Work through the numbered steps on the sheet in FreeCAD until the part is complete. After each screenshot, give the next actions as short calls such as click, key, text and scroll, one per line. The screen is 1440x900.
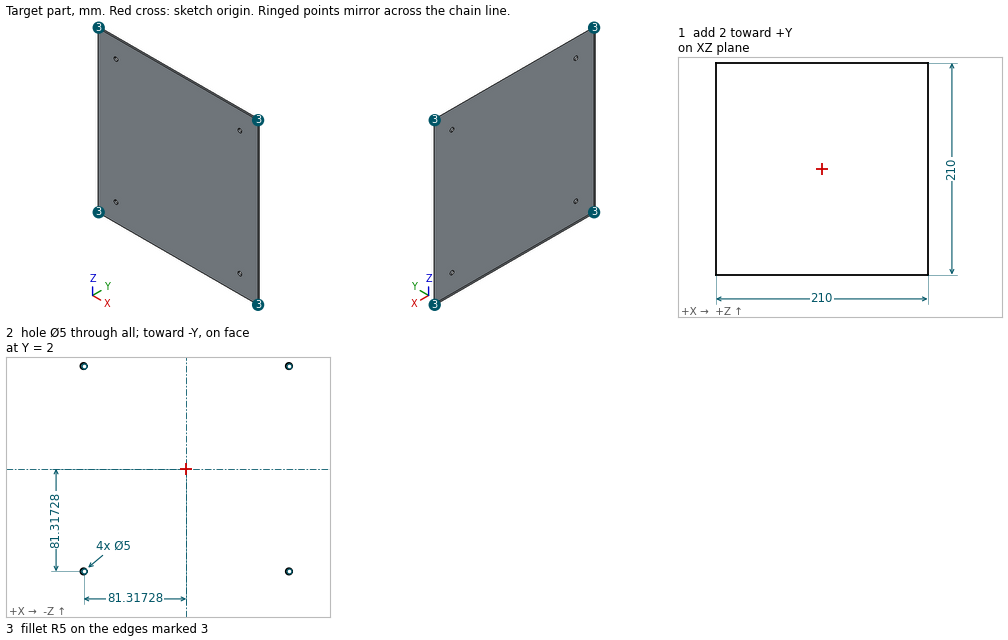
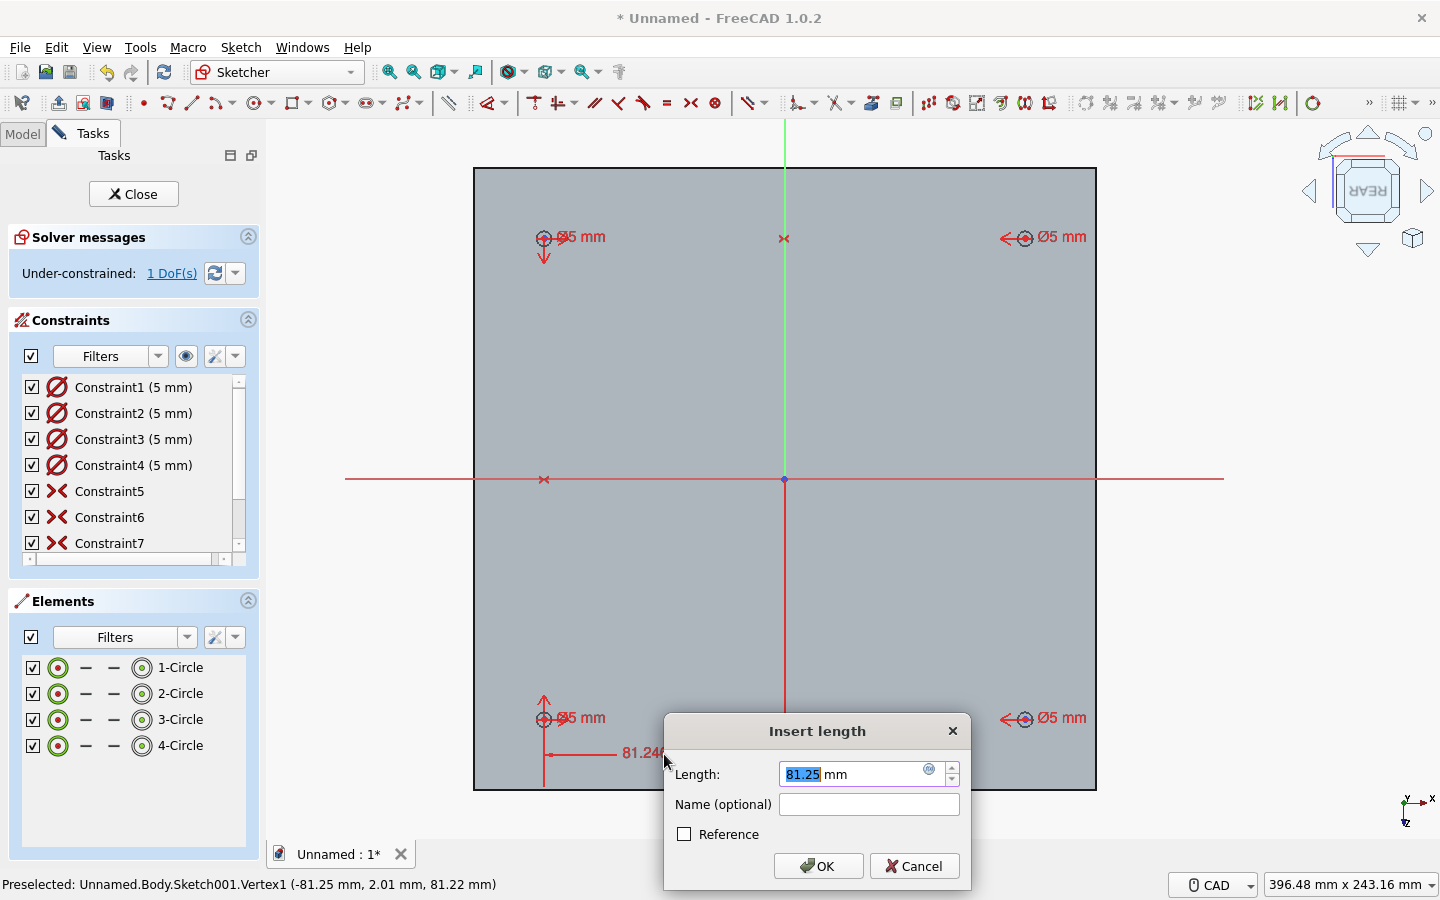
text(81.31728)
key(Return)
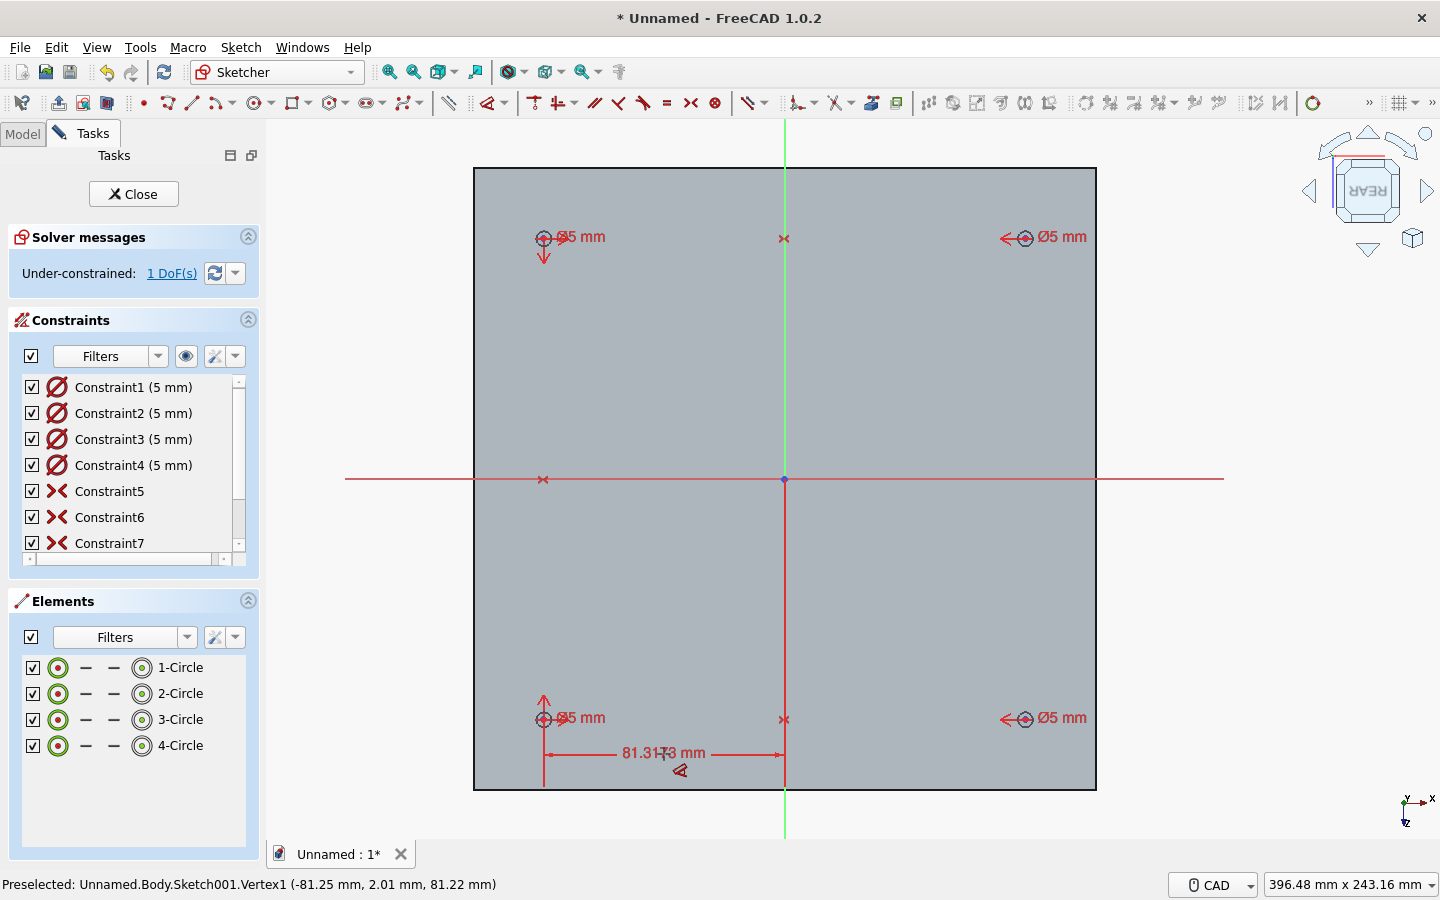
click(544, 720)
click(510, 600)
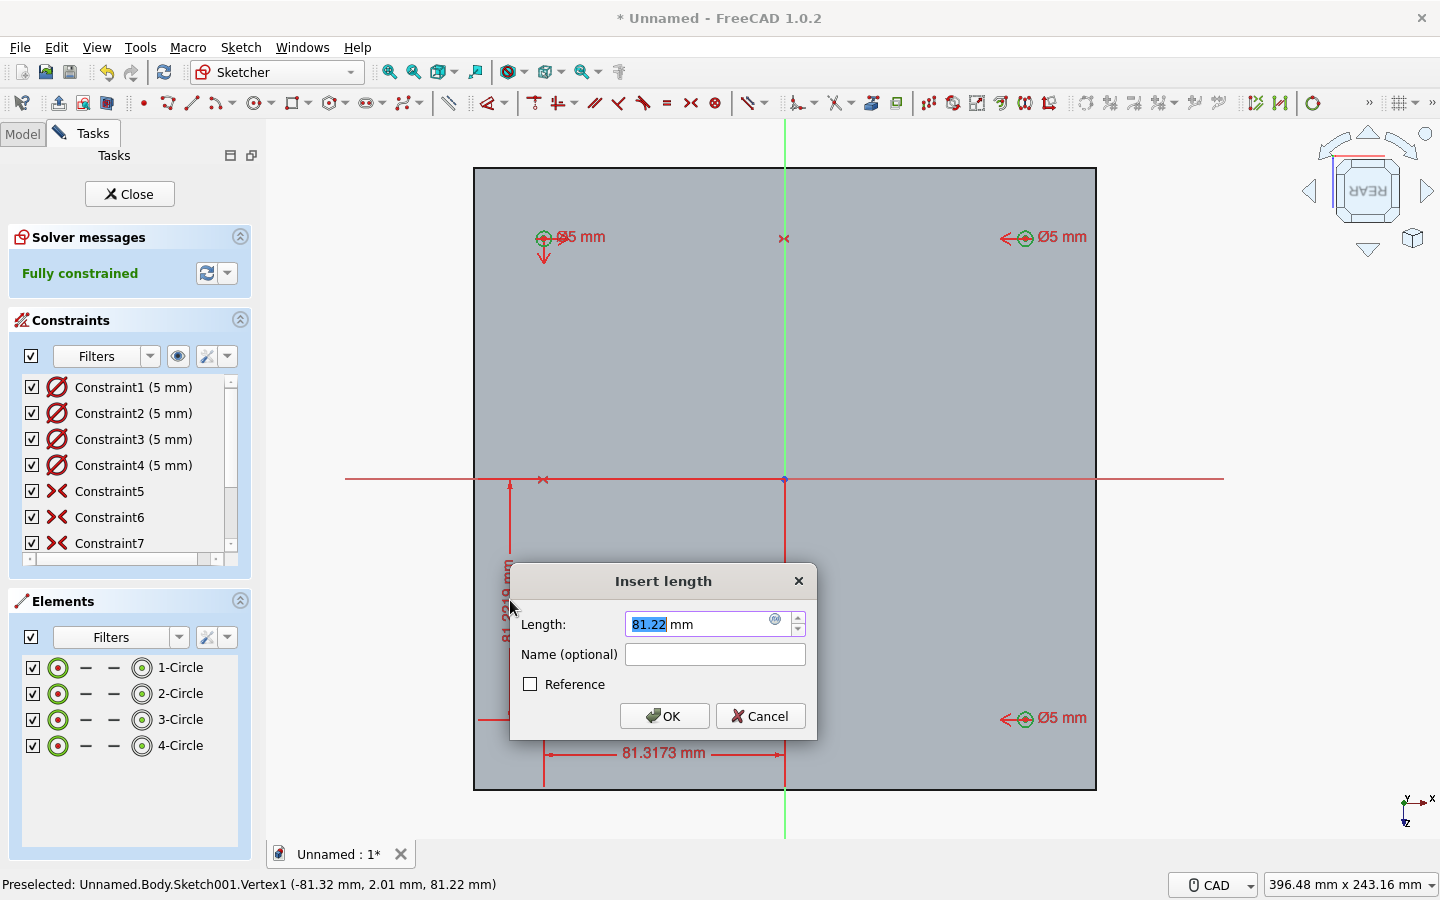
text(81.31728)
key(Return)
key(Escape)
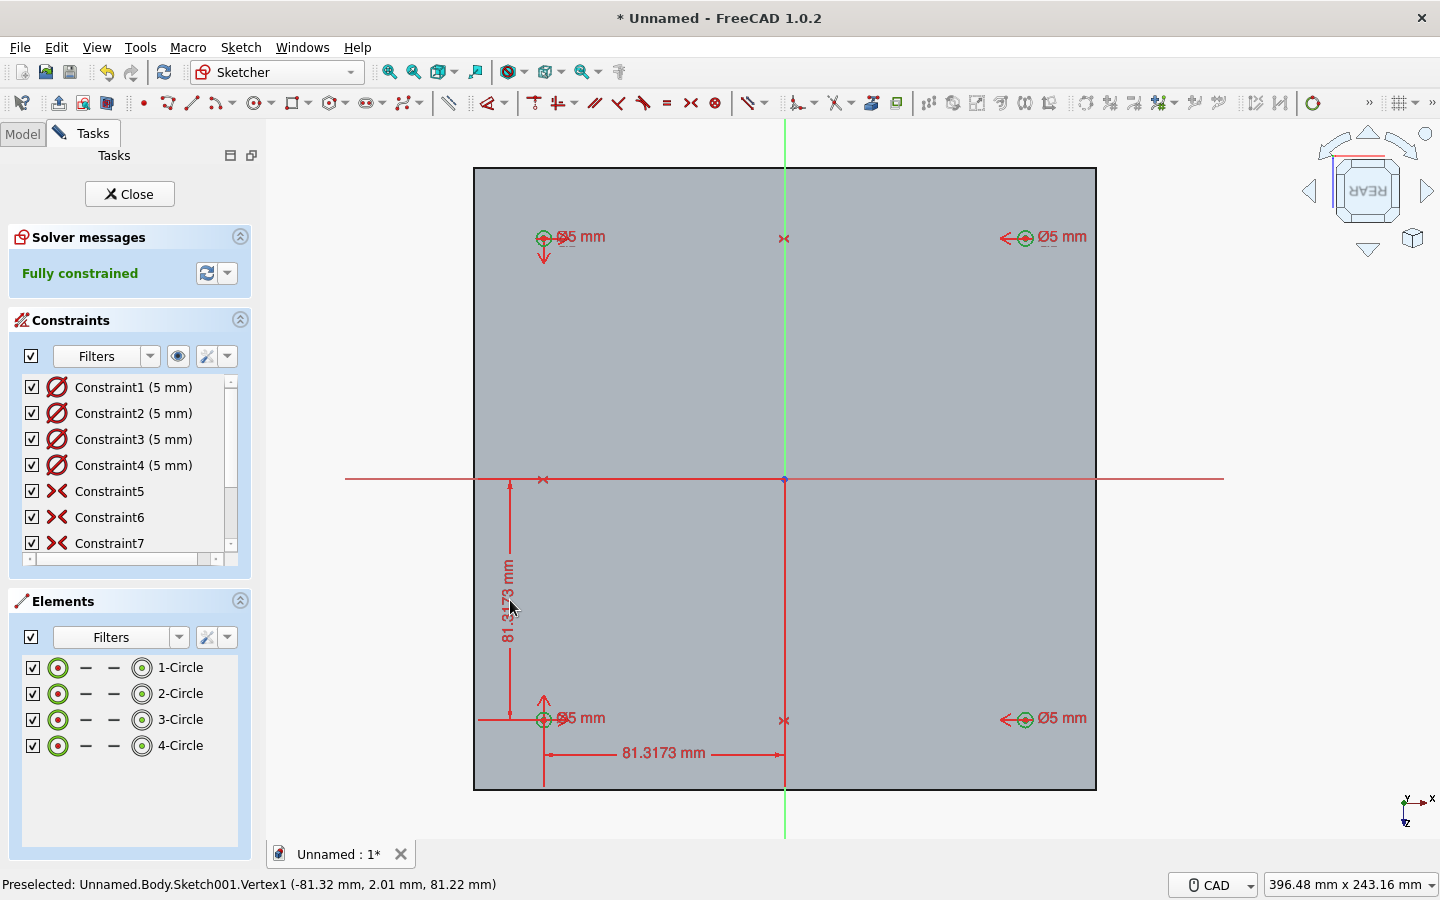
click(130, 194)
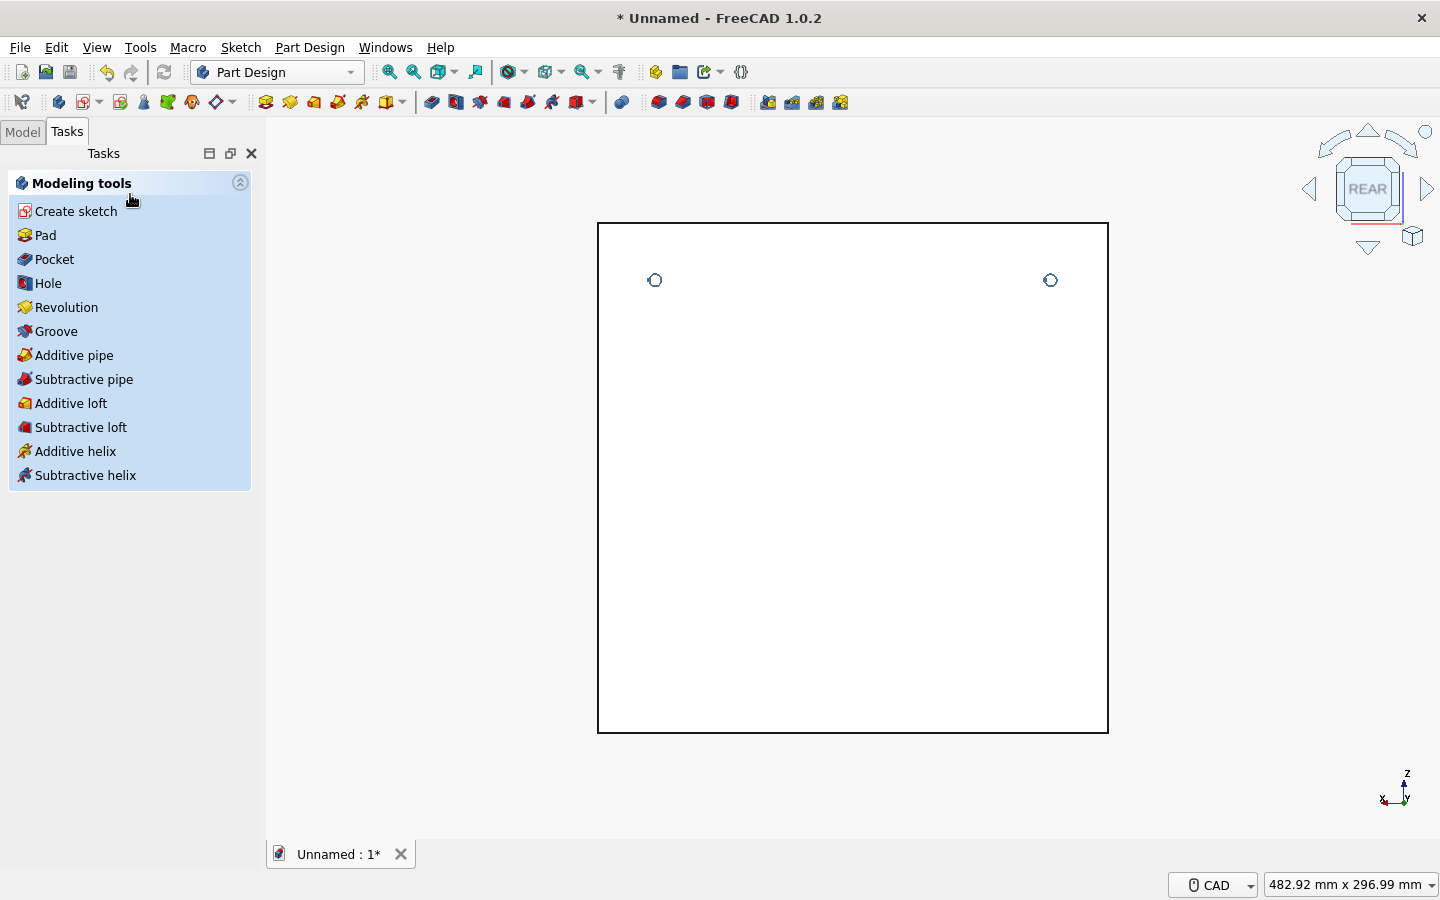
click(456, 102)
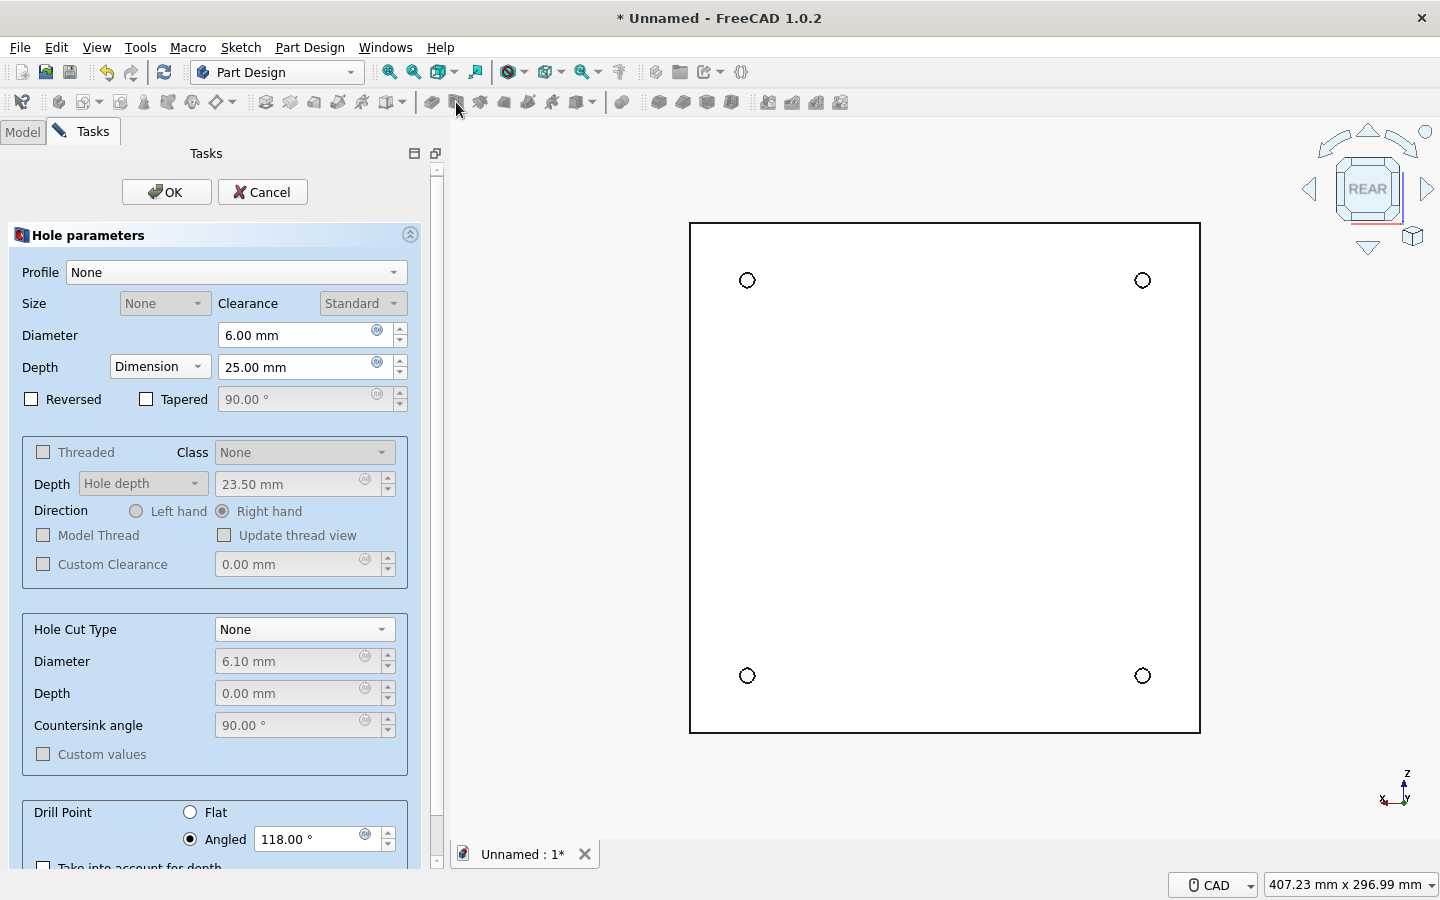
triple_click(305, 335)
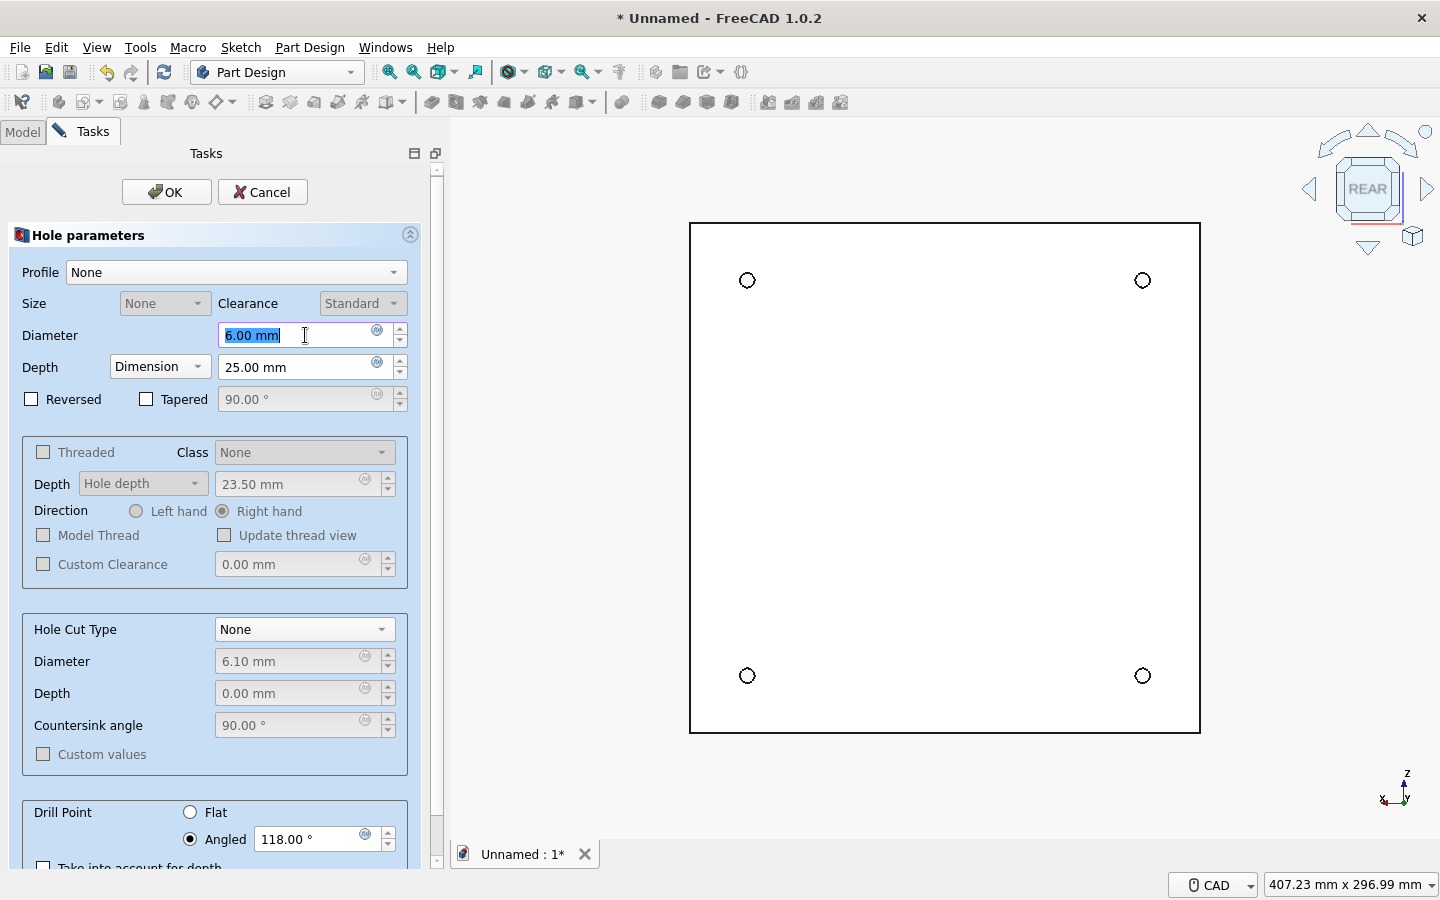
text(5)
key(Tab)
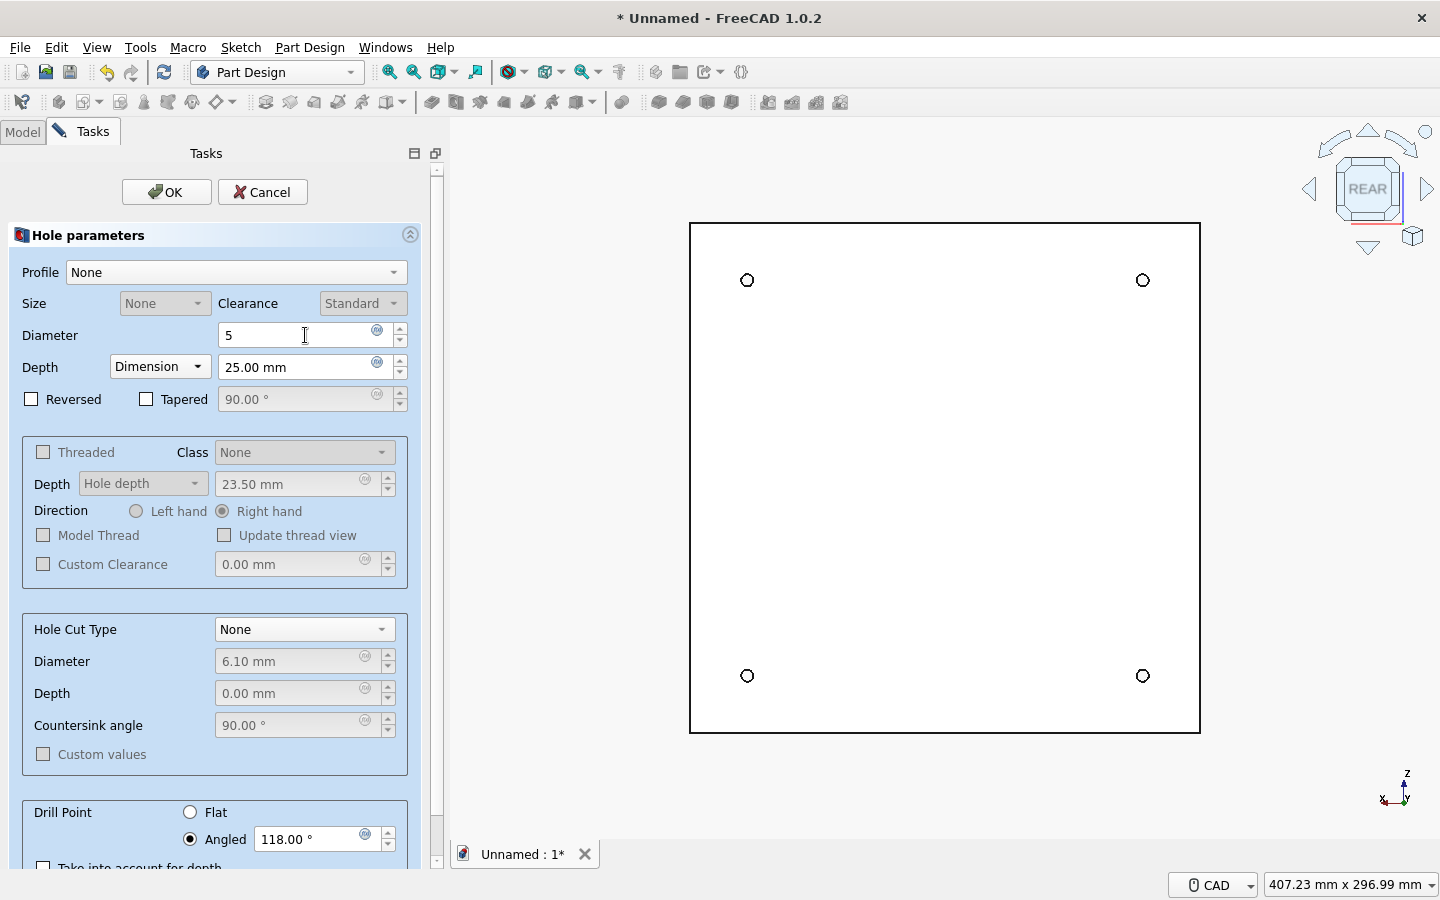
click(161, 366)